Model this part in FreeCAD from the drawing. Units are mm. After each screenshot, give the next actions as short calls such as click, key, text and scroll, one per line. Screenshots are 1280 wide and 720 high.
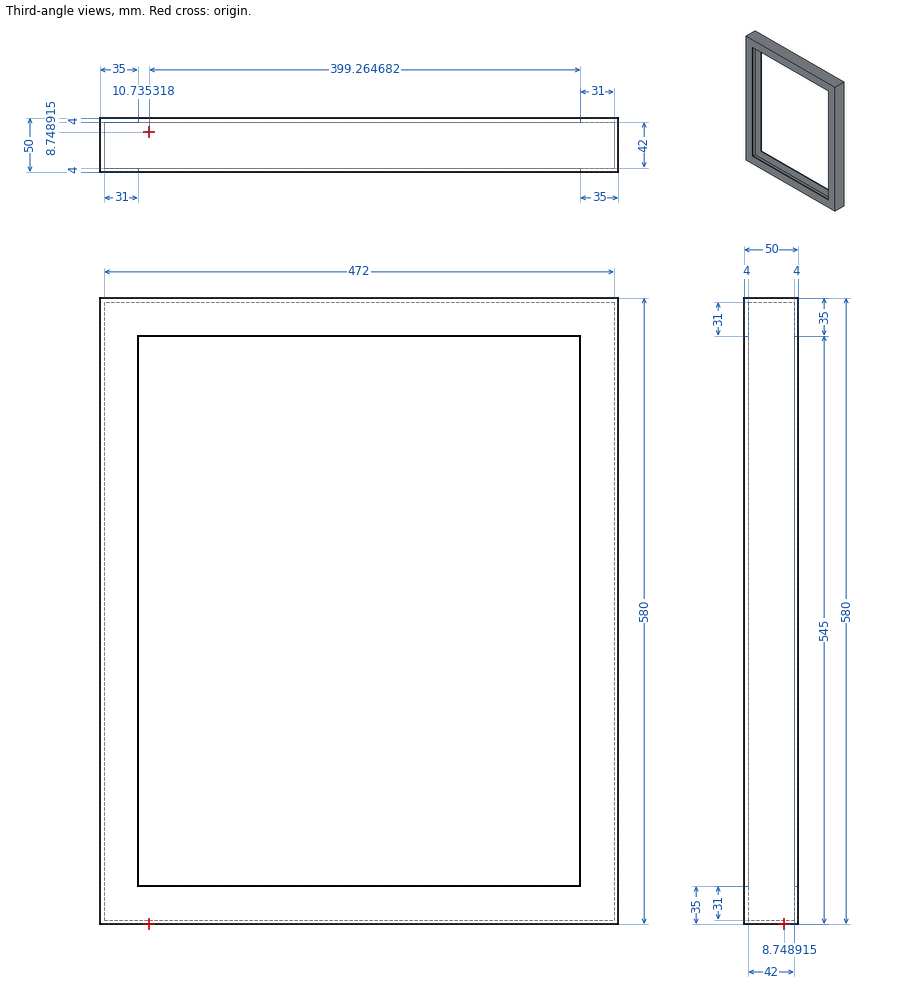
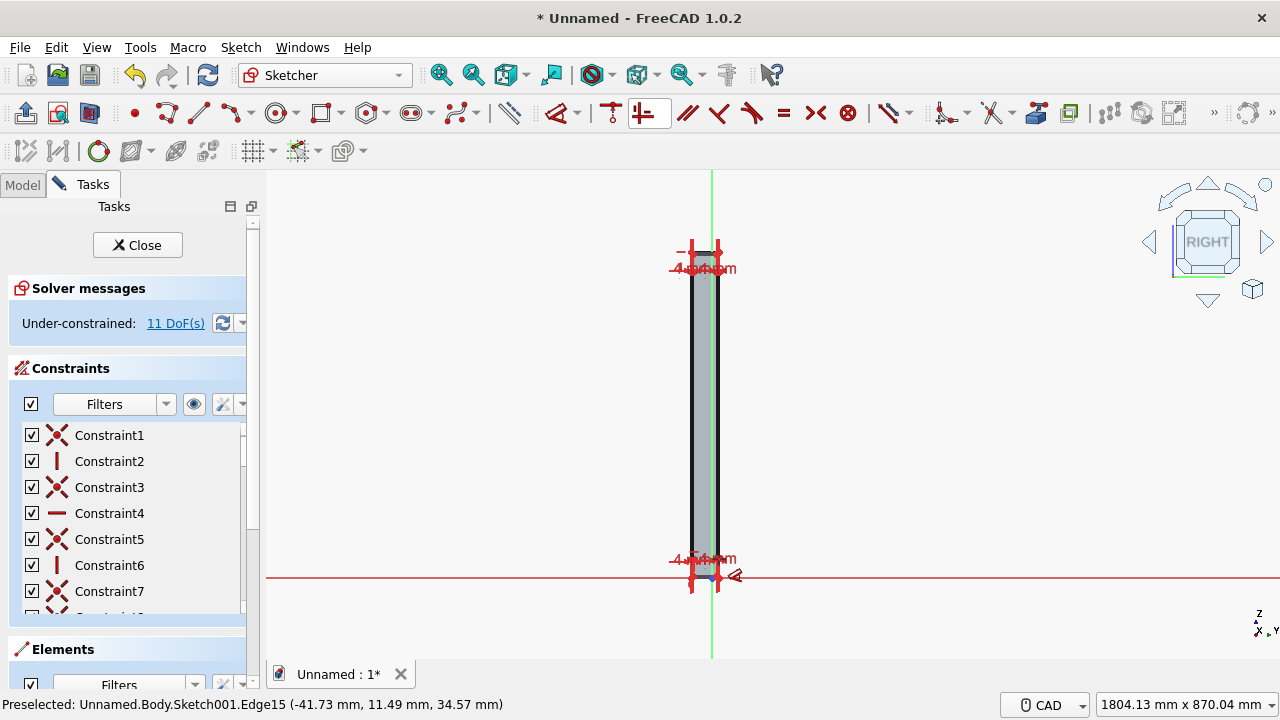
scroll(719, 266, up, 10)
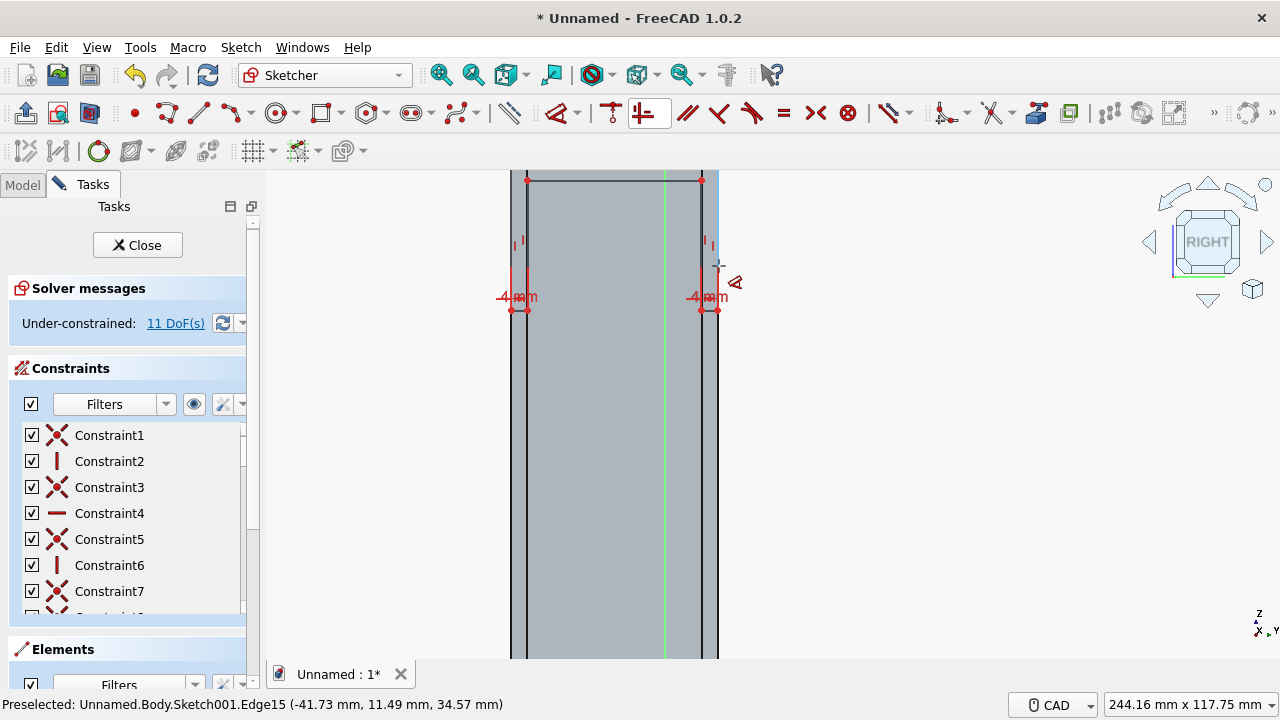
click(718, 268)
click(752, 254)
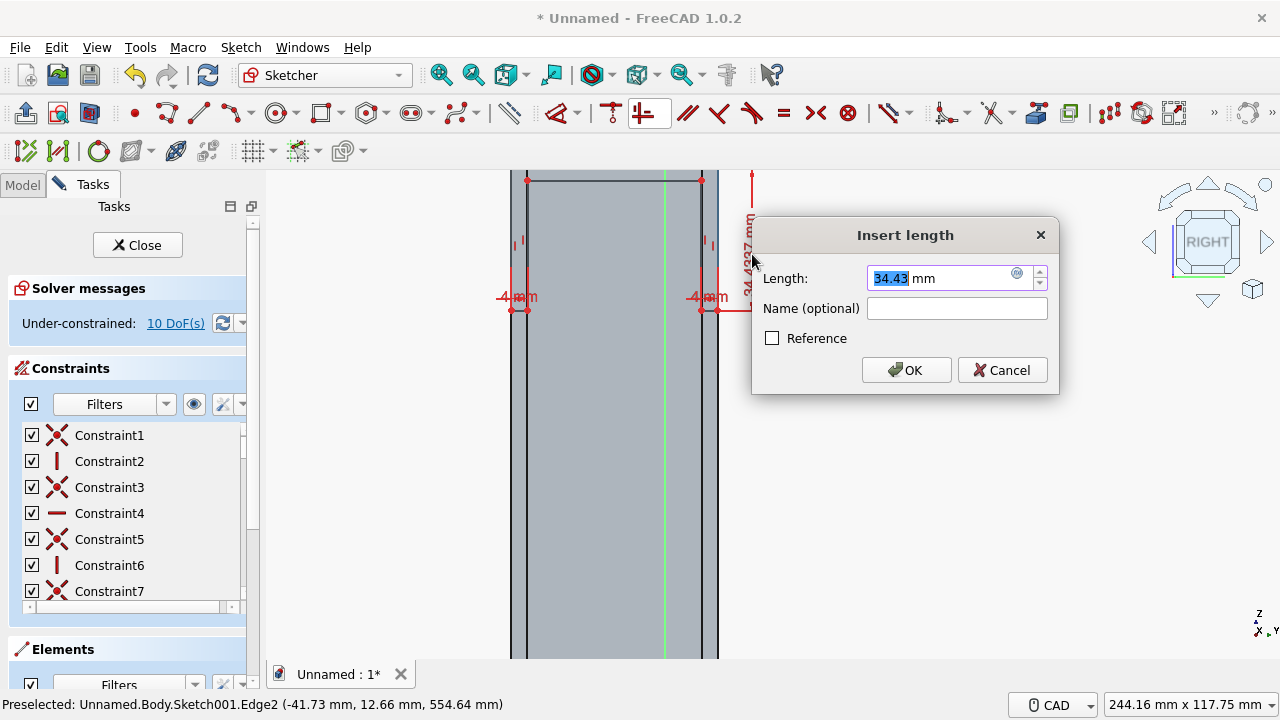
text(35)
key(Return)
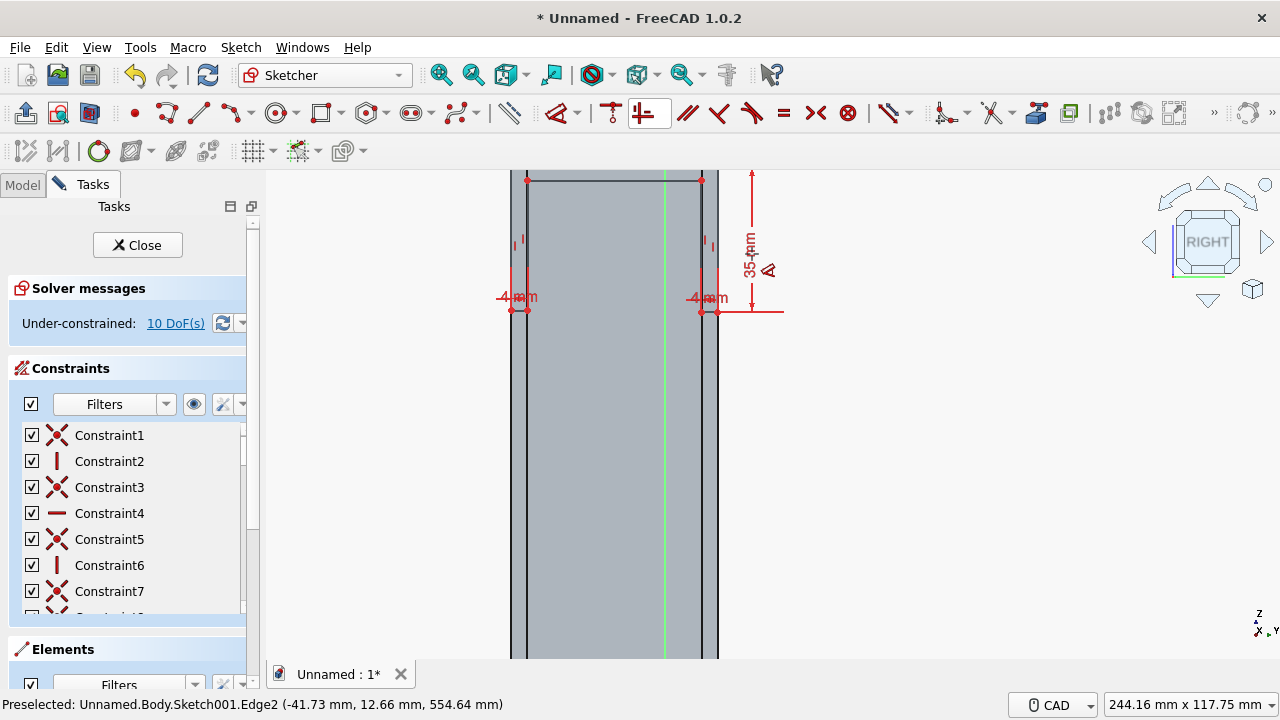
scroll(719, 265, down, 10)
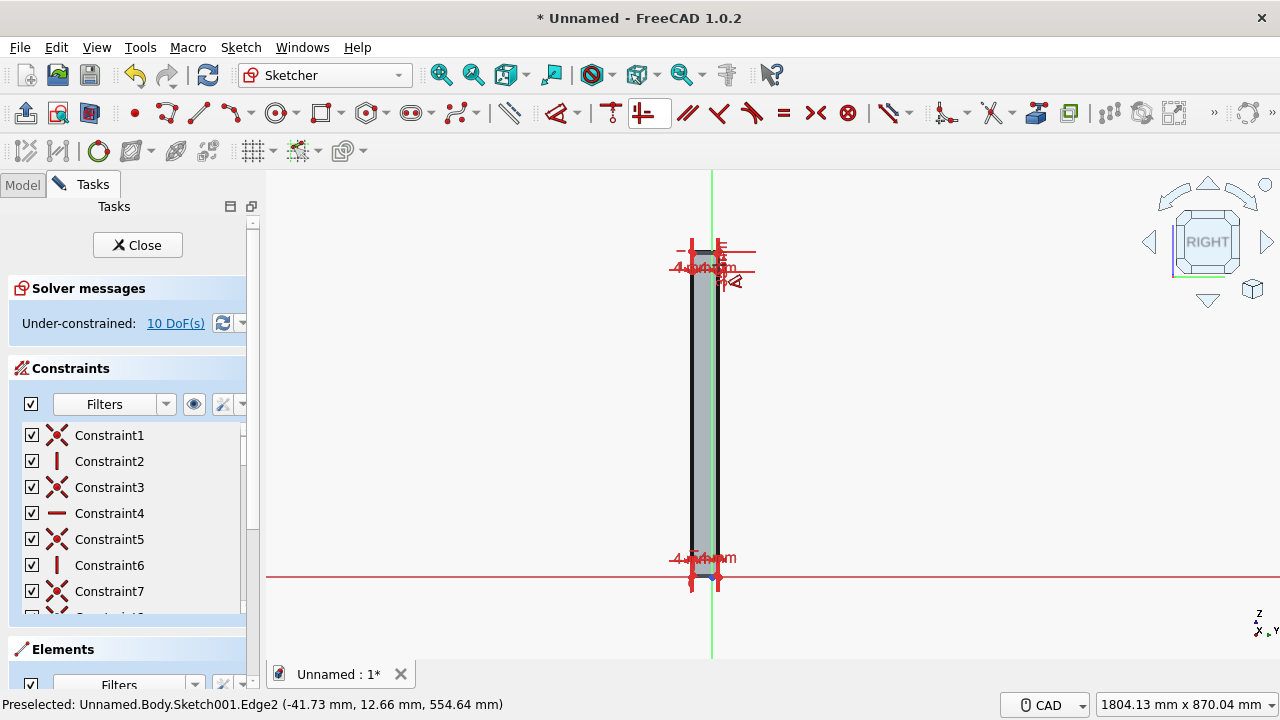
scroll(711, 252, up, 12)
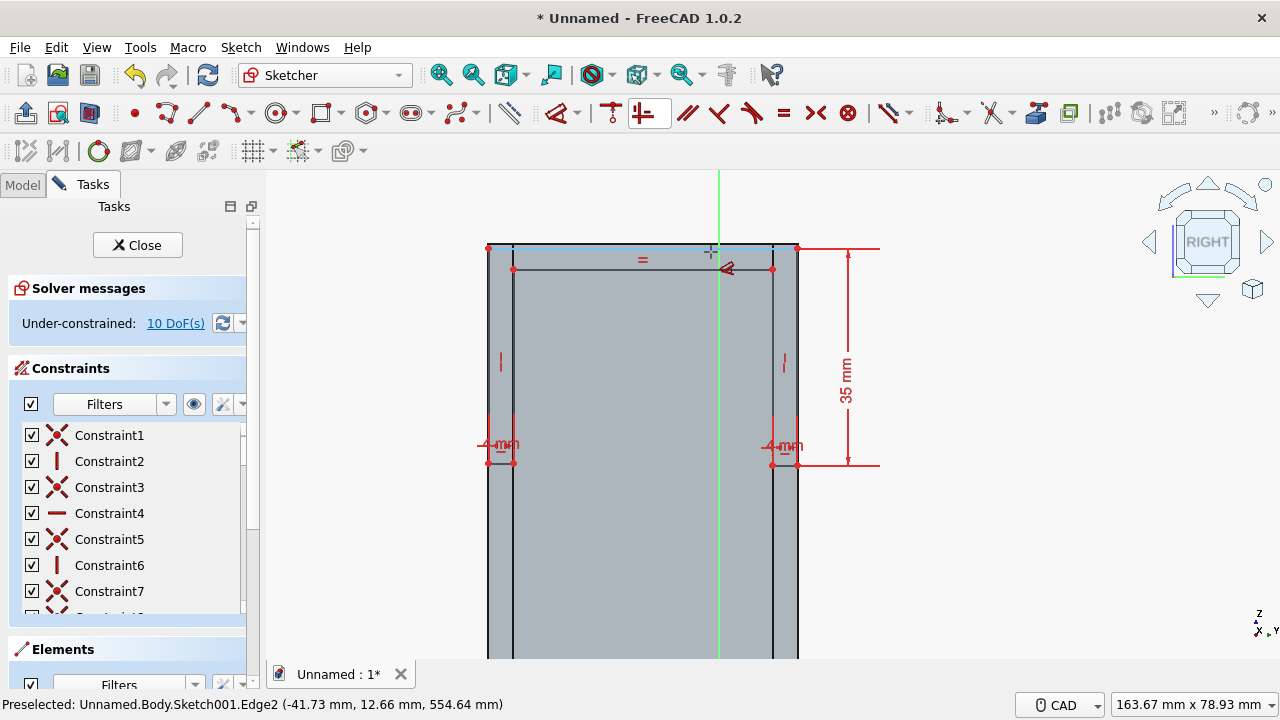
click(705, 249)
click(643, 215)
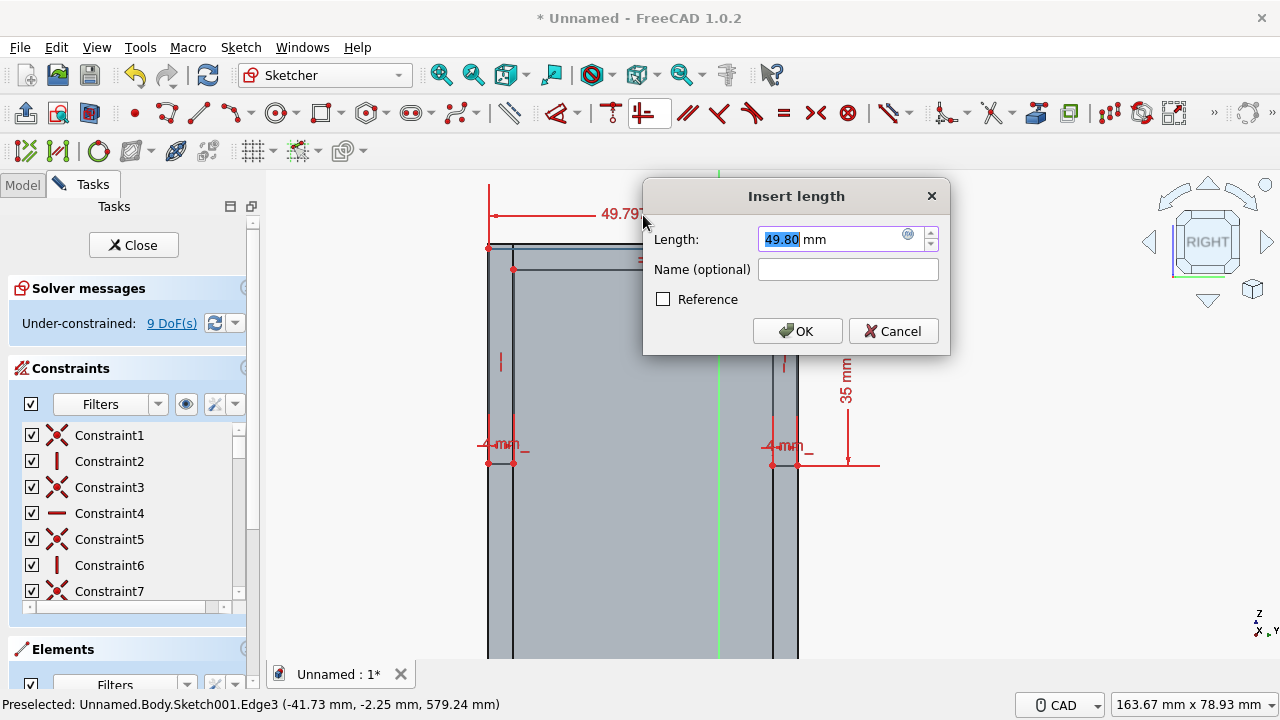
text(50)
key(Return)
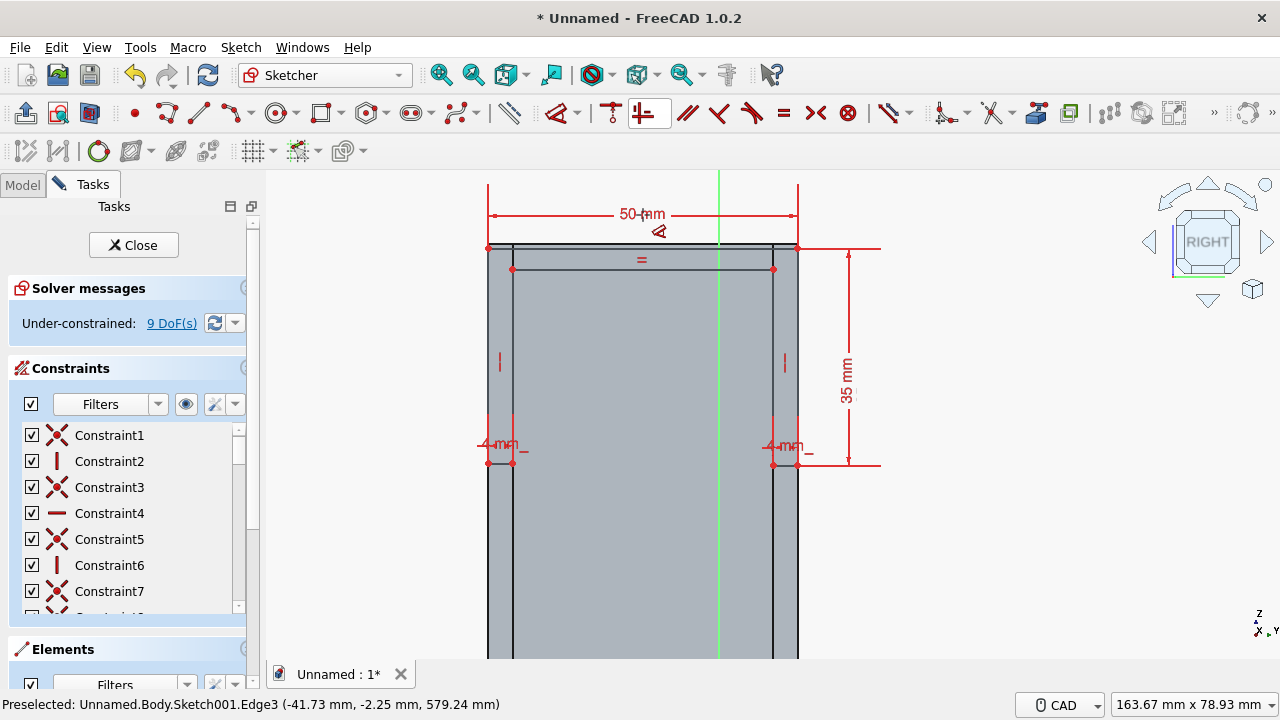
click(488, 313)
click(454, 356)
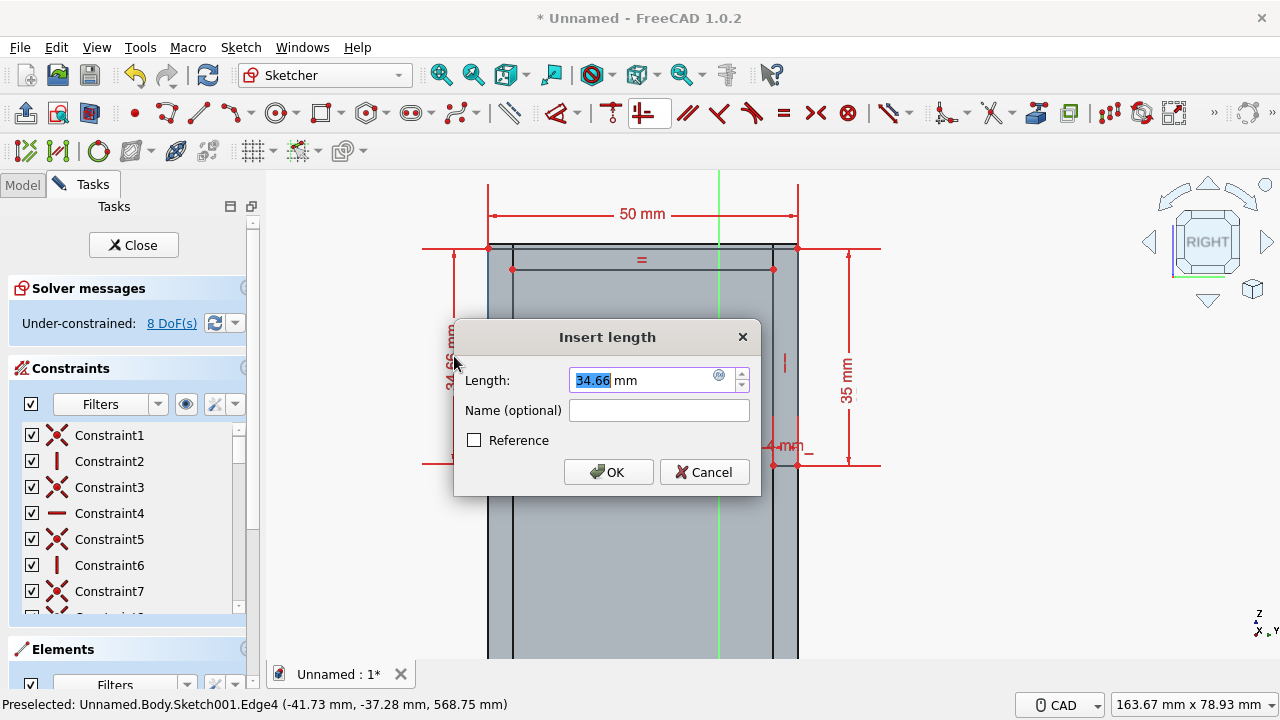
text(35)
key(Return)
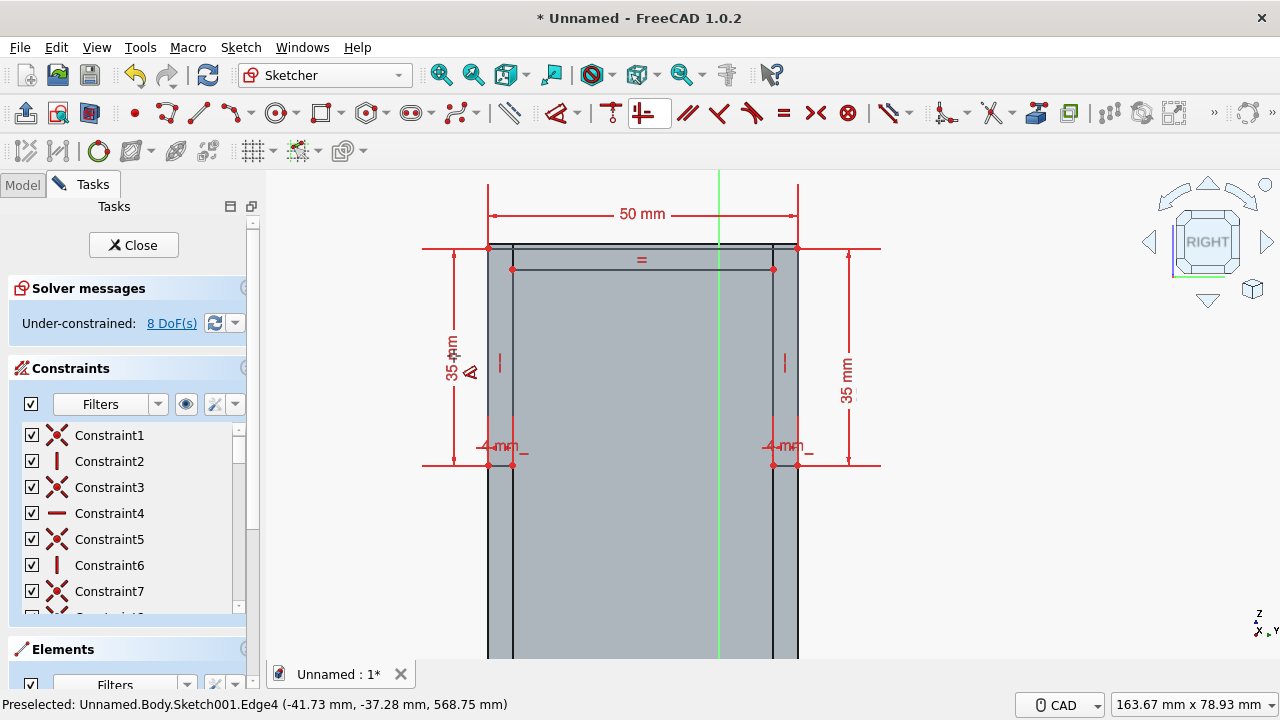
click(513, 407)
click(547, 368)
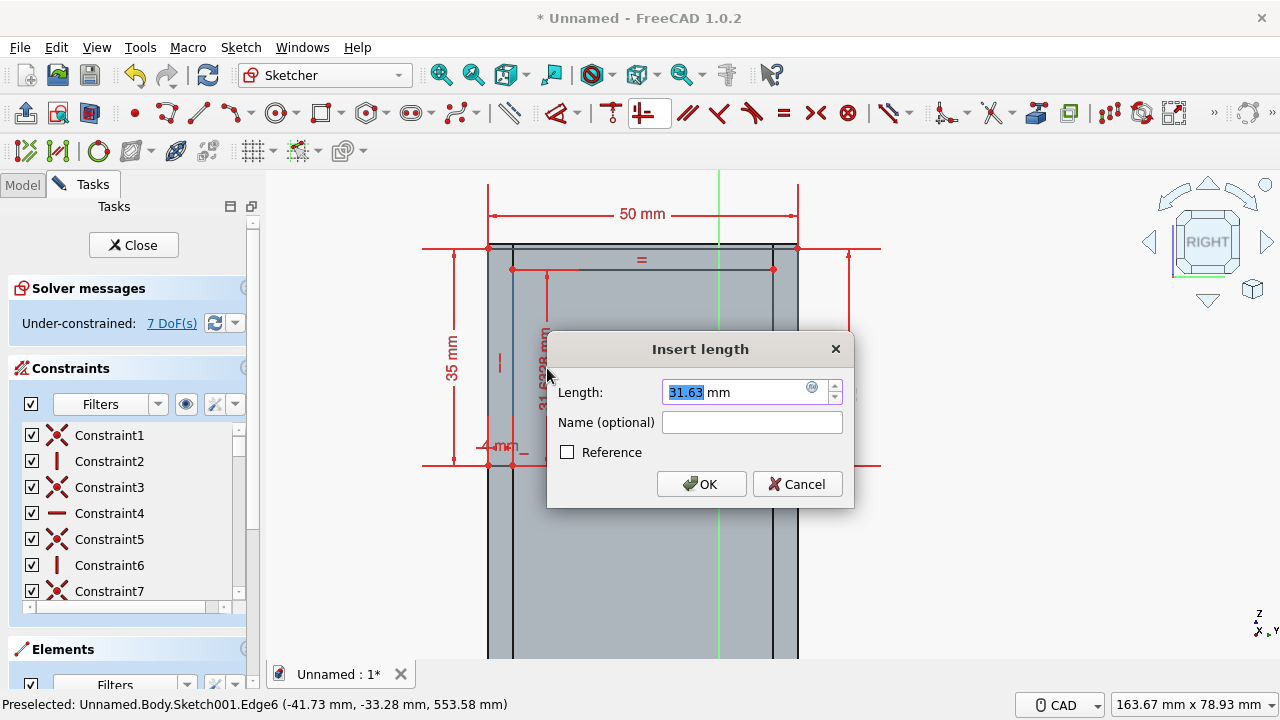
text(31)
key(Return)